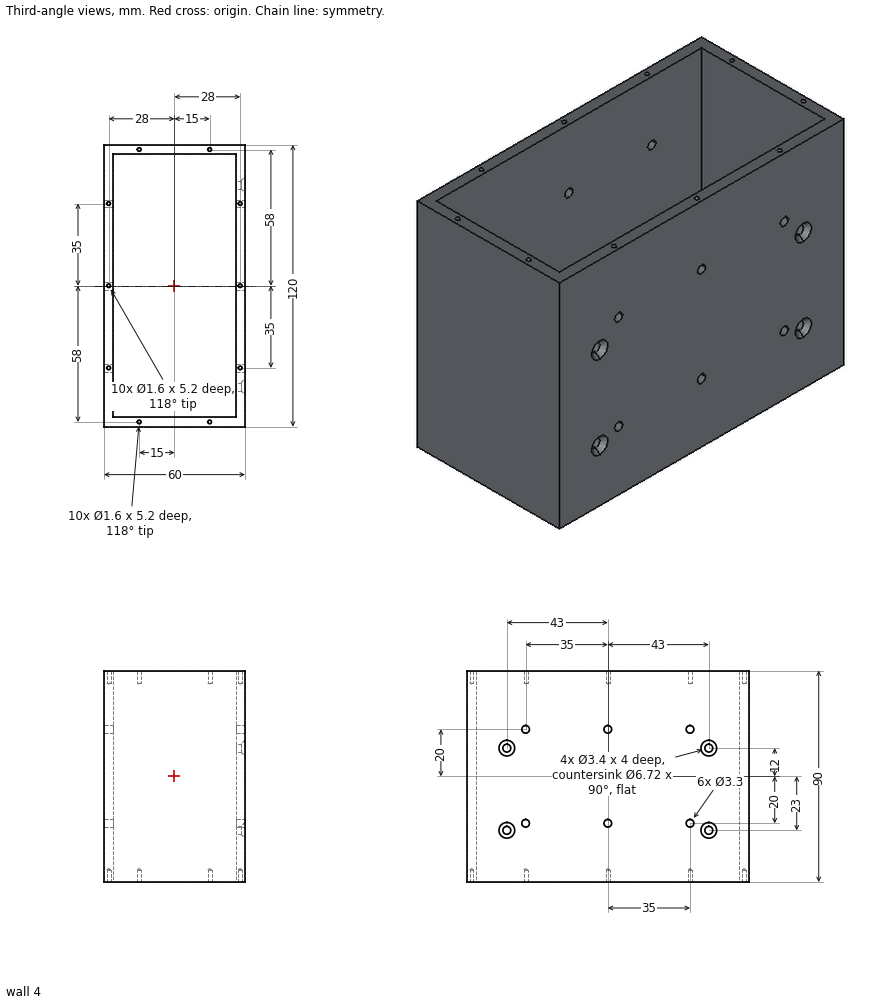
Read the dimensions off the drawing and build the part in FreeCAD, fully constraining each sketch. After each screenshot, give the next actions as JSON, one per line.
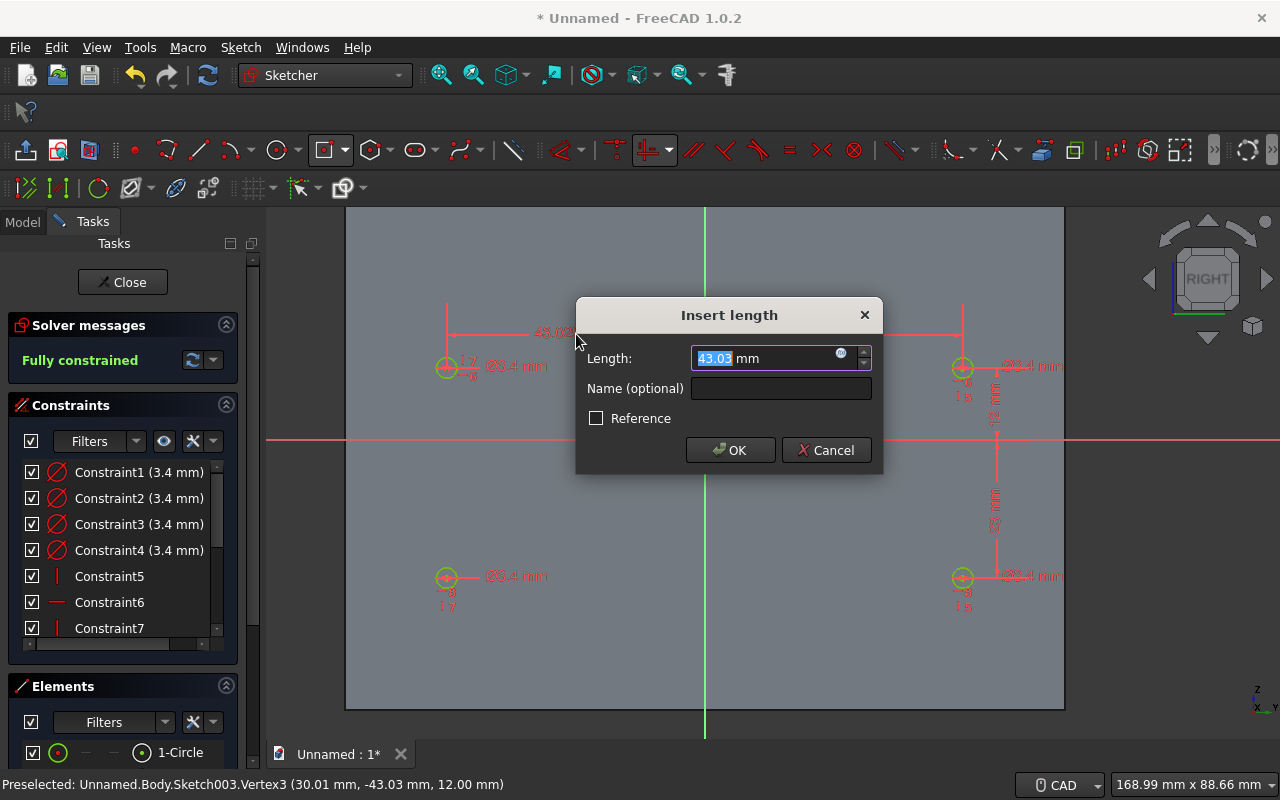
{"action": "type", "text": "43"}
{"action": "key", "text": "Return"}
{"action": "key", "text": "Escape"}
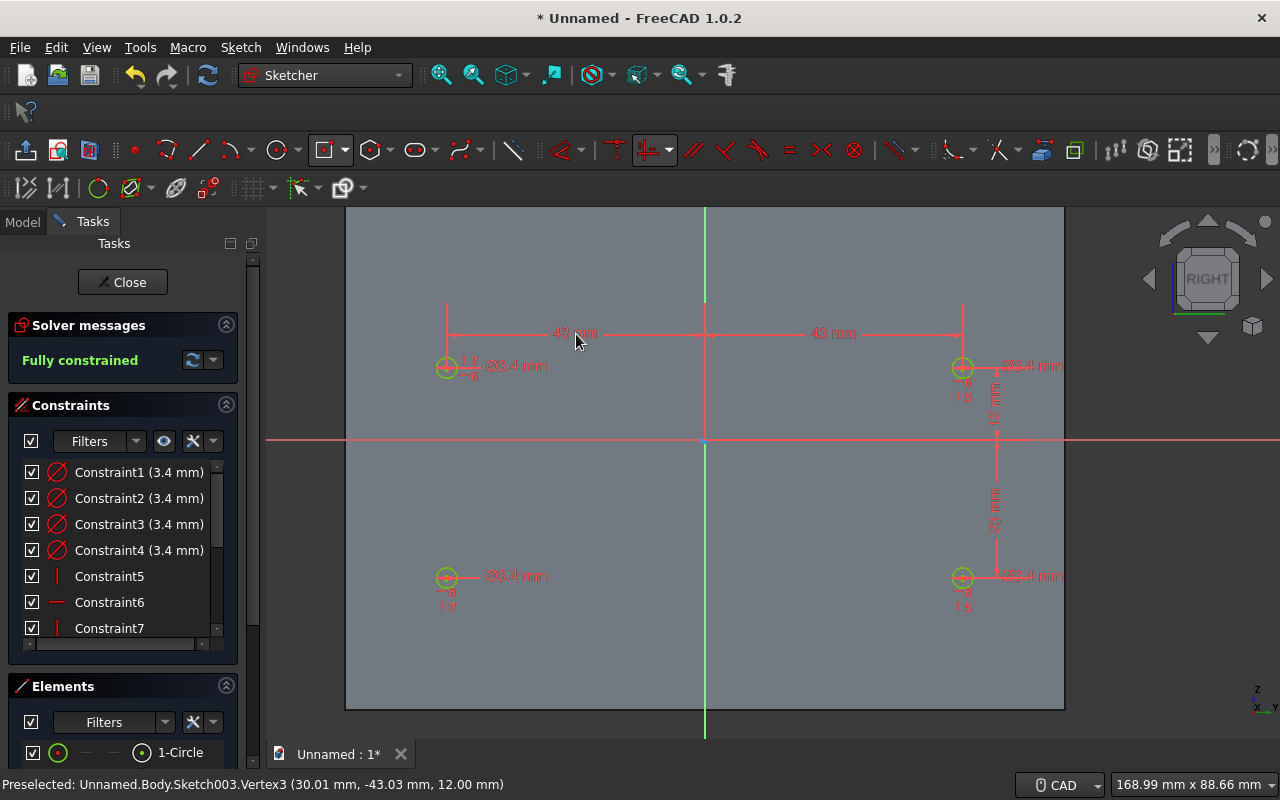
{"action": "left_click", "coordinate": [123, 282]}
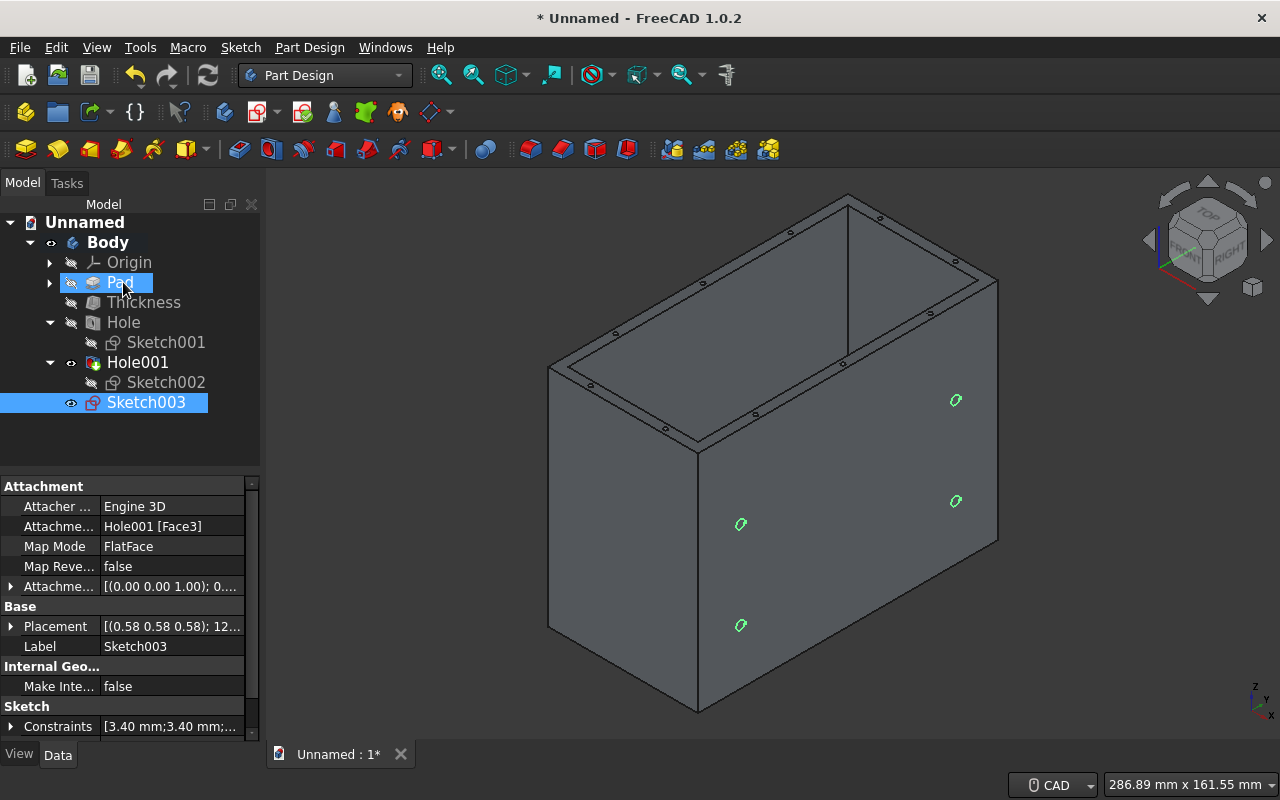
{"action": "left_click", "coordinate": [272, 150]}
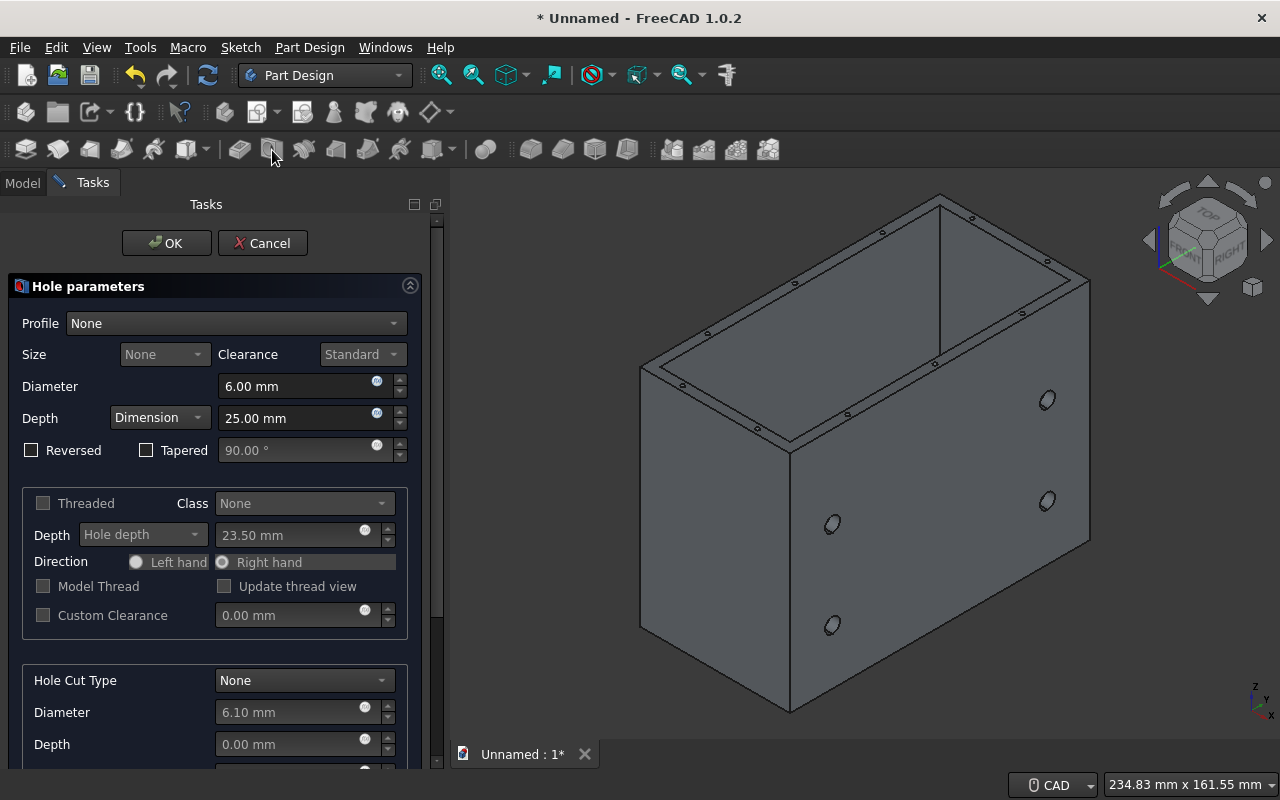
{"action": "triple_click", "coordinate": [305, 386]}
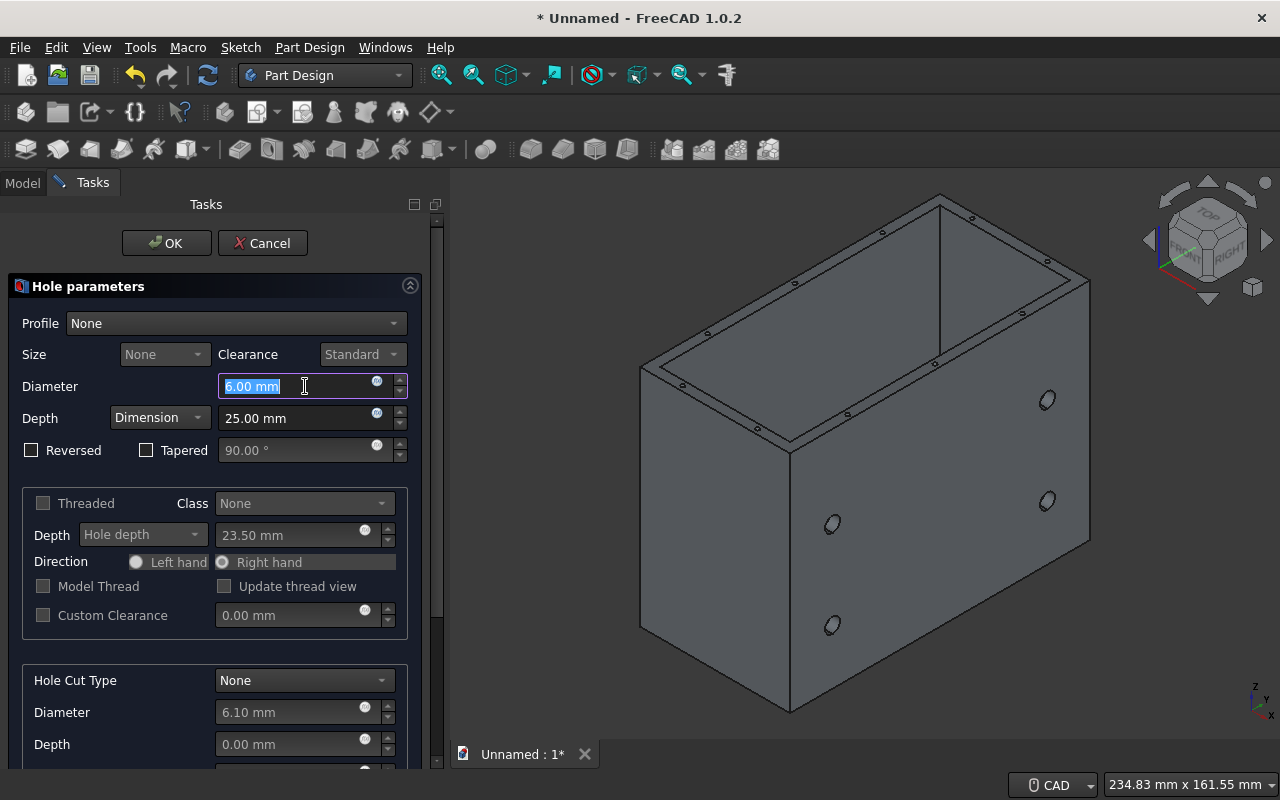
{"action": "type", "text": "3.4"}
{"action": "key", "text": "Tab"}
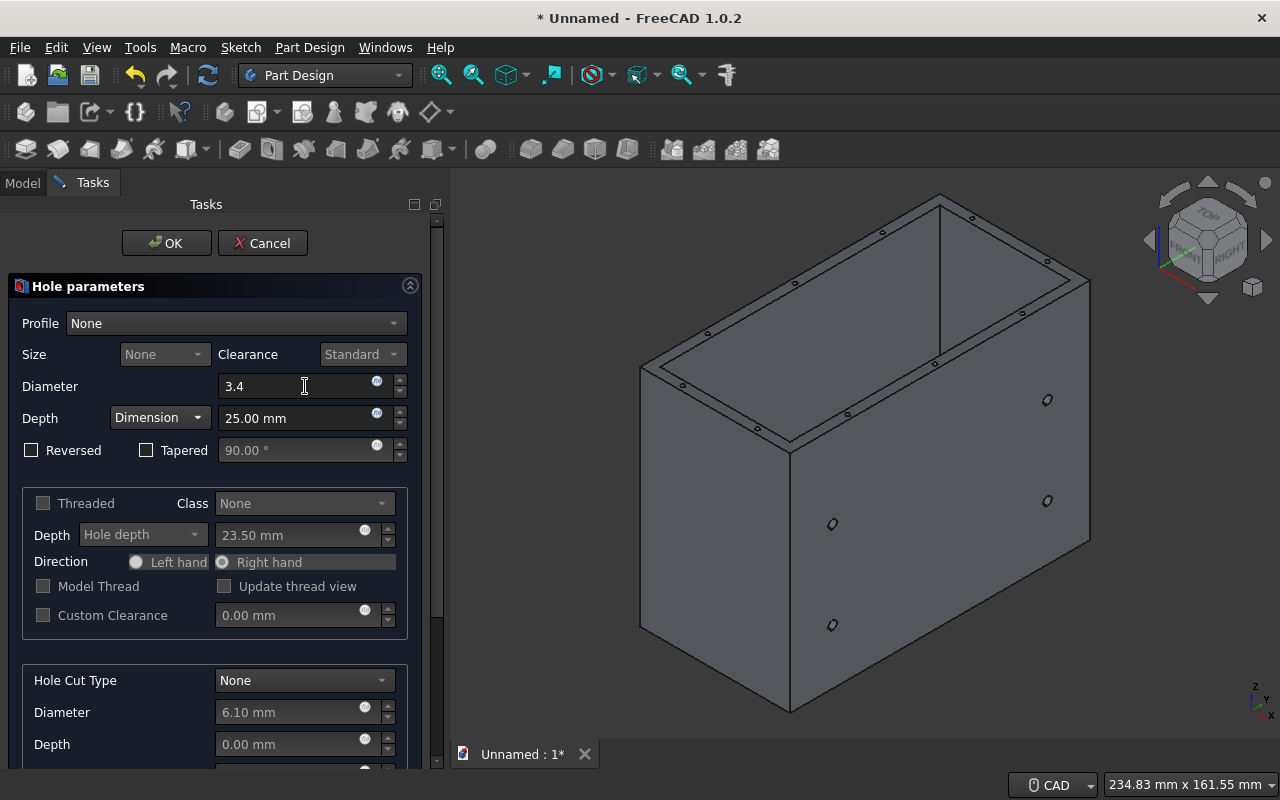
{"action": "triple_click", "coordinate": [305, 418]}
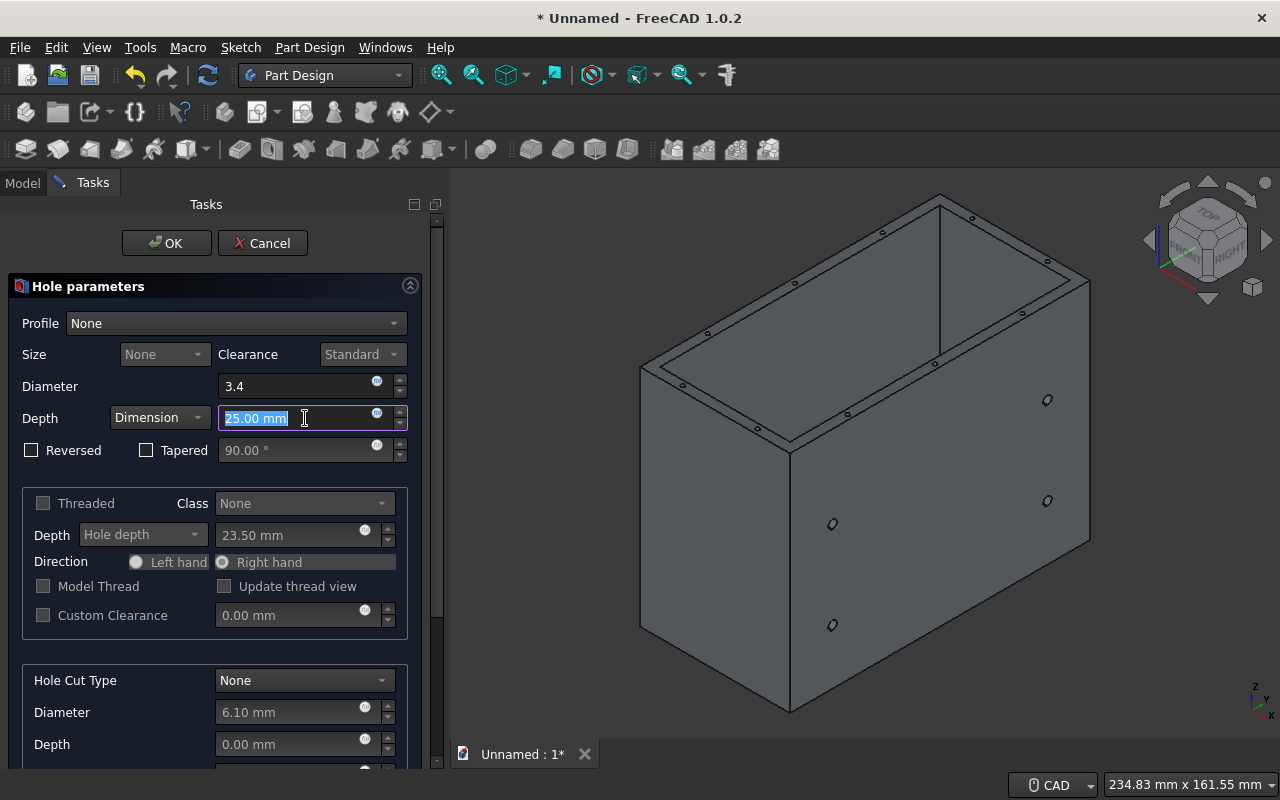
{"action": "type", "text": "4"}
{"action": "key", "text": "Tab"}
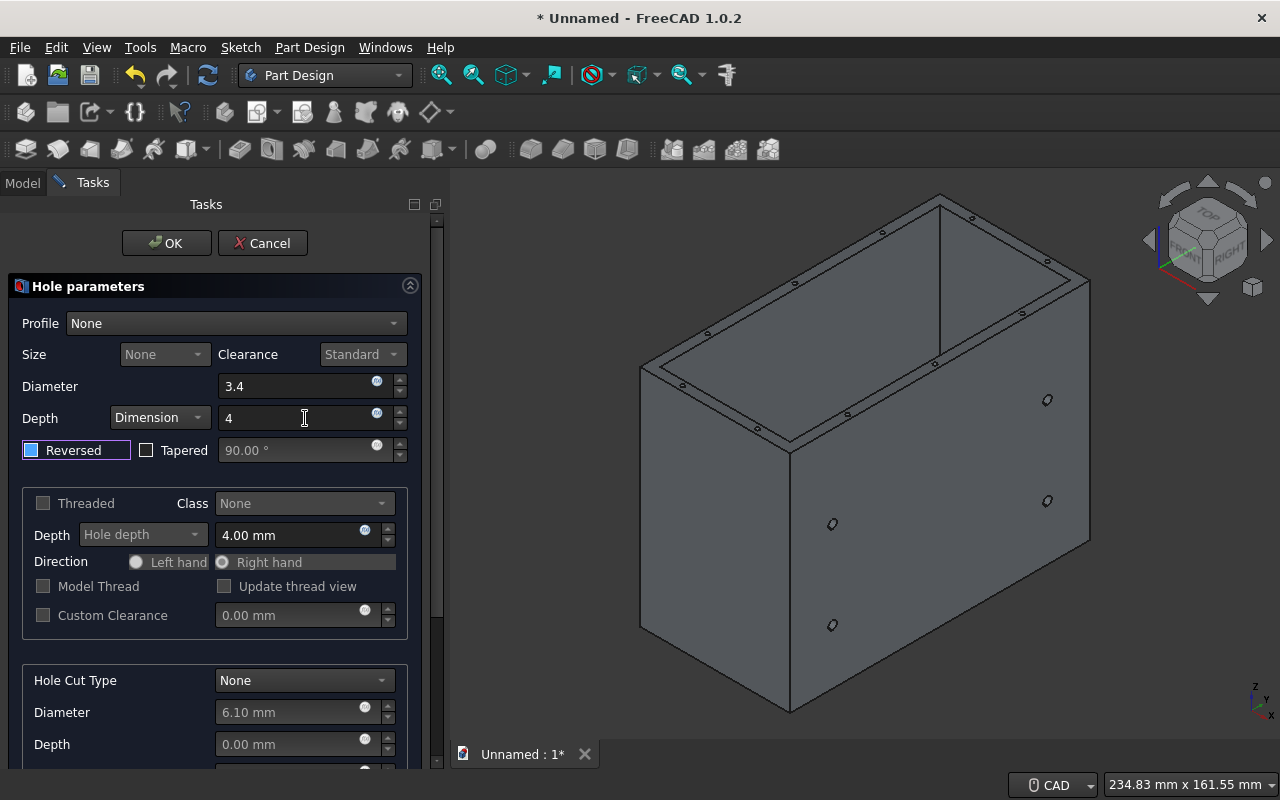
{"action": "left_click", "coordinate": [306, 680]}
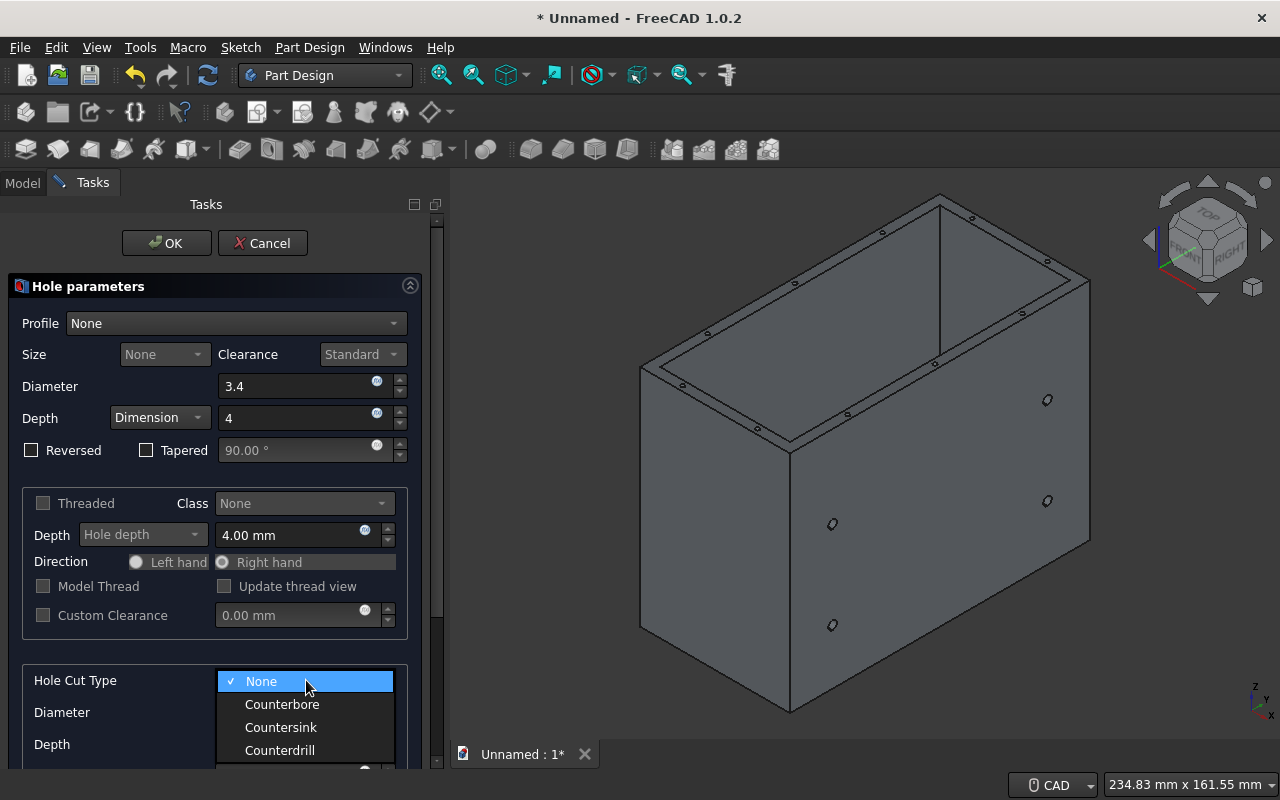
{"action": "left_click", "coordinate": [304, 728]}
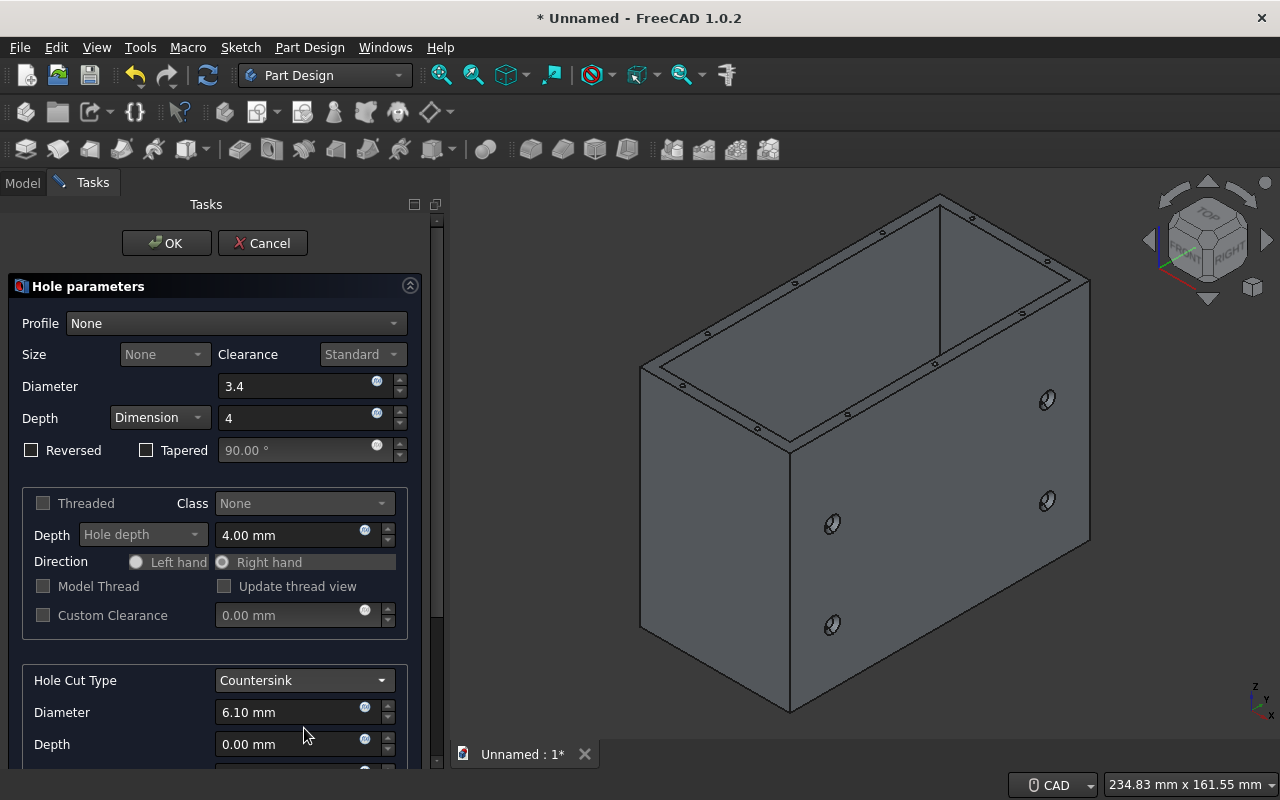
{"action": "triple_click", "coordinate": [298, 712]}